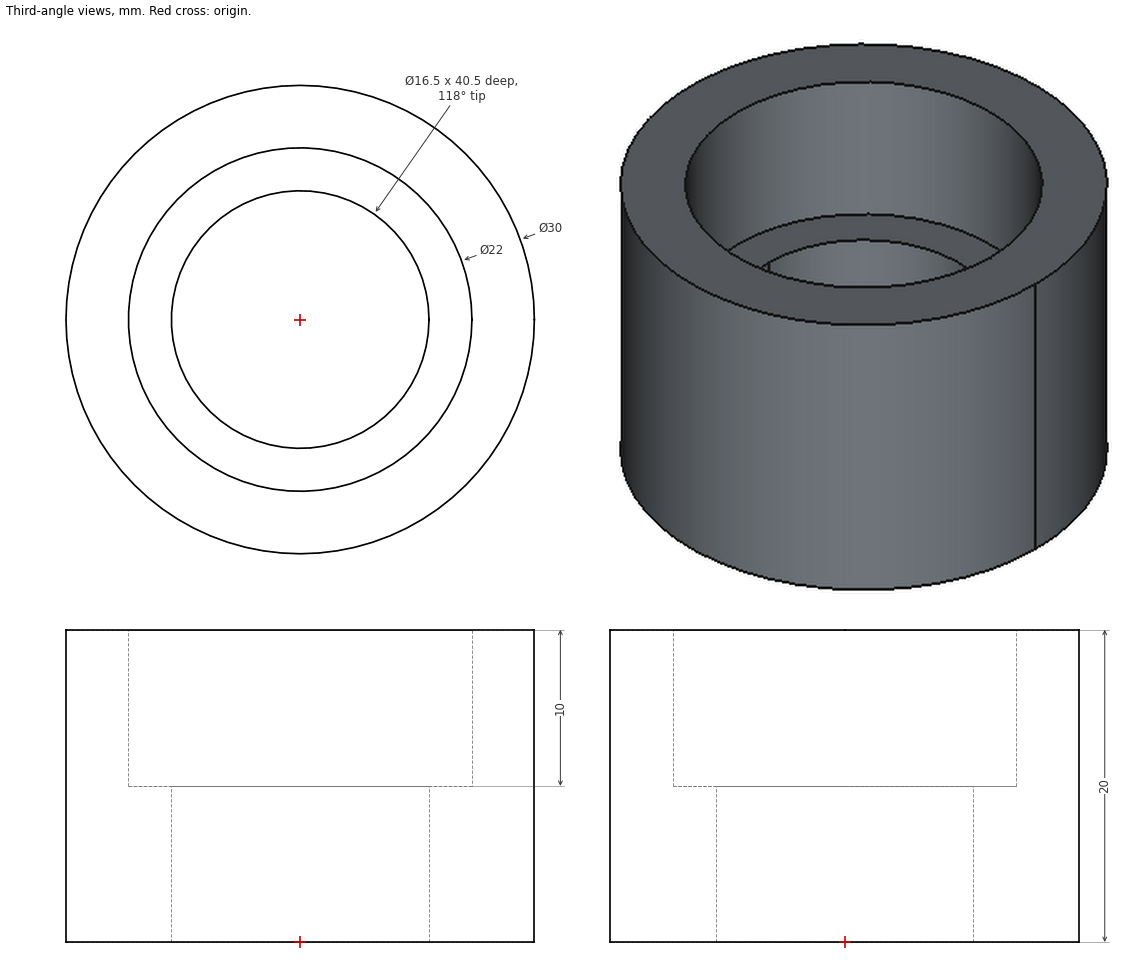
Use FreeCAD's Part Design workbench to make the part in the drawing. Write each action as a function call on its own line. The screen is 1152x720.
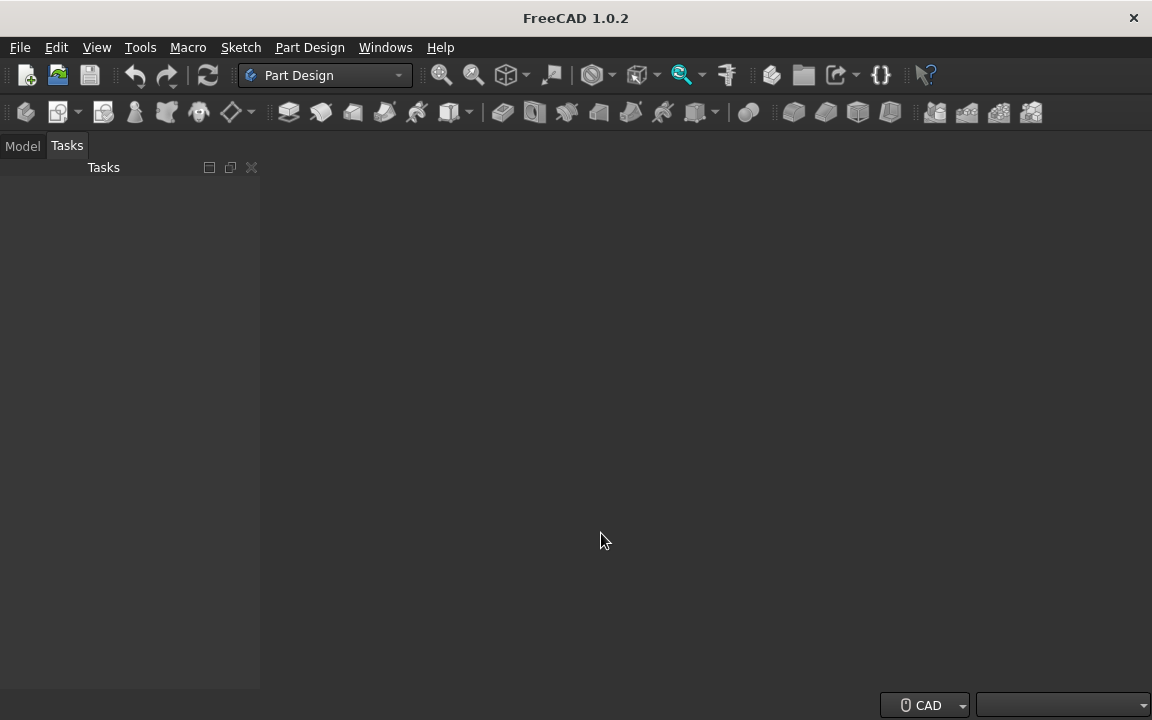
click(26, 76)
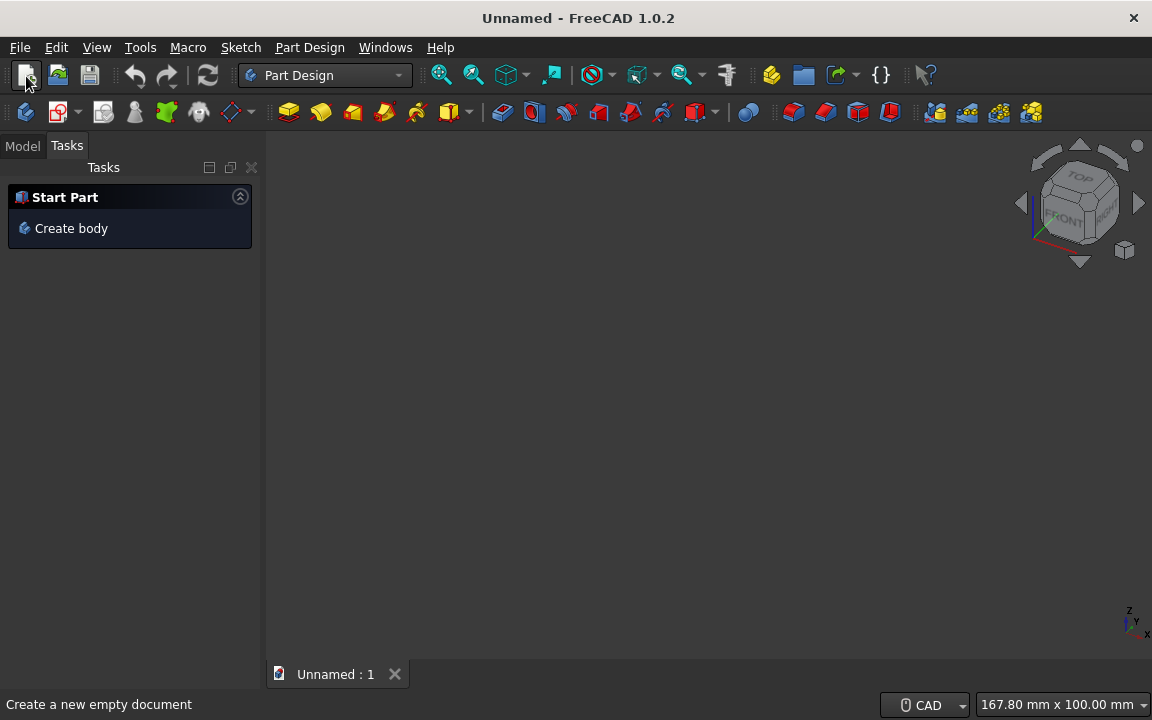
click(58, 112)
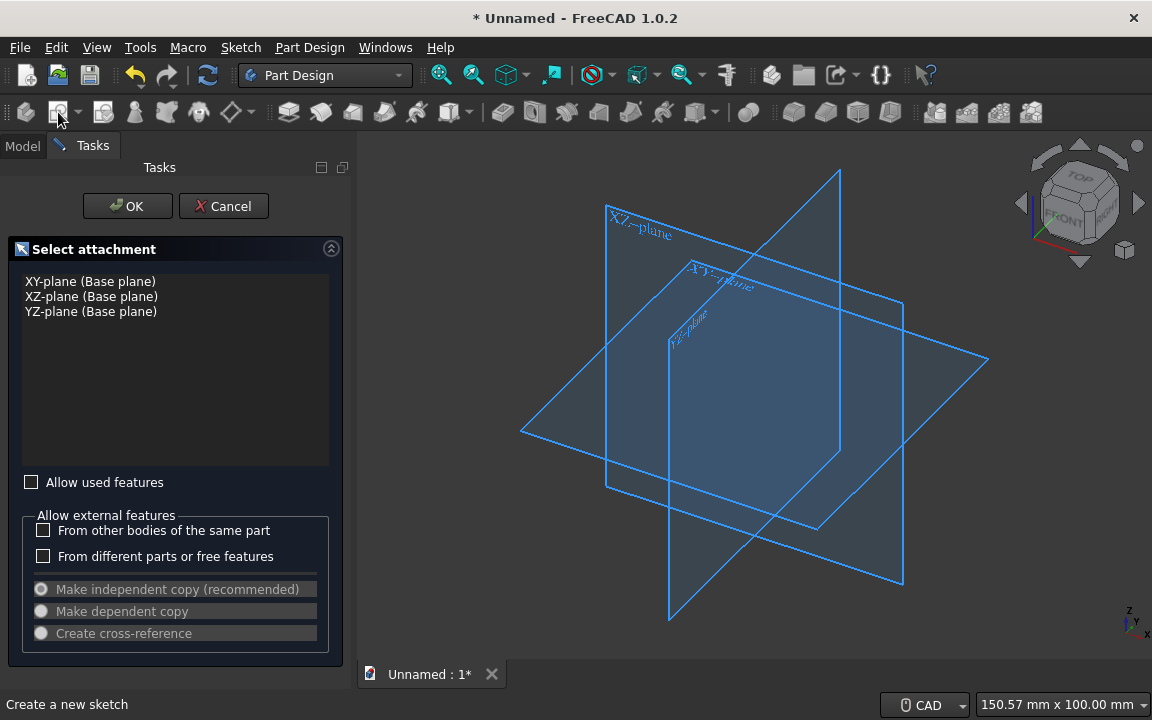
click(82, 282)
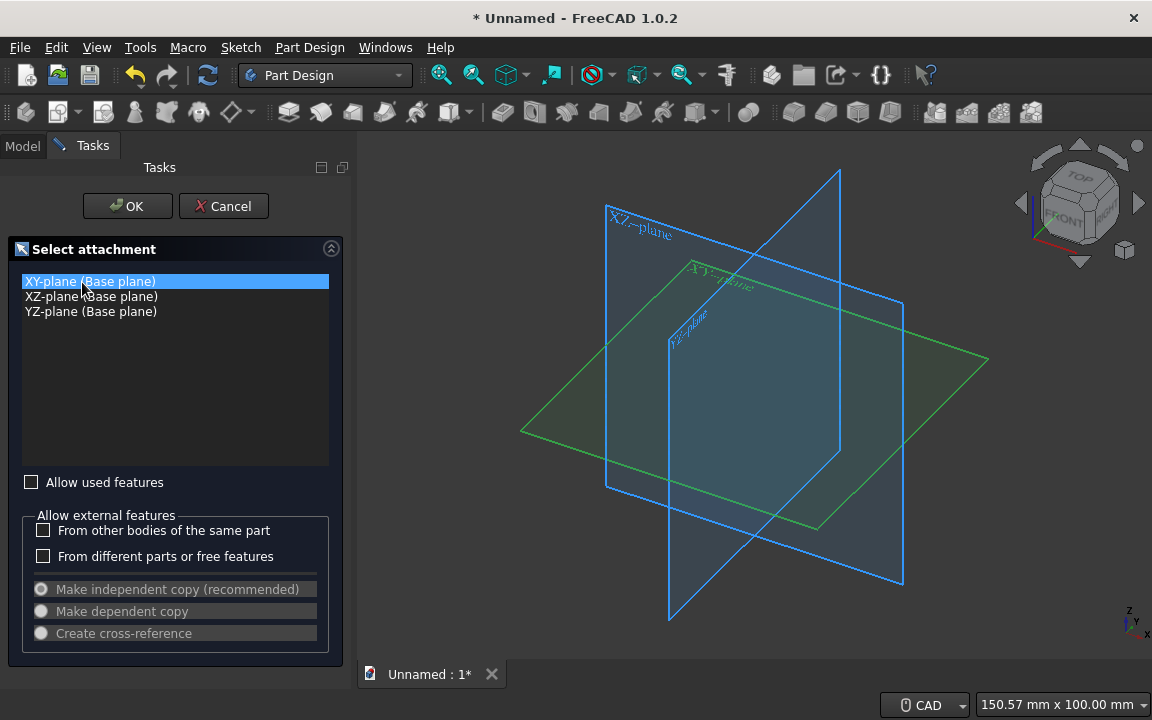
click(128, 206)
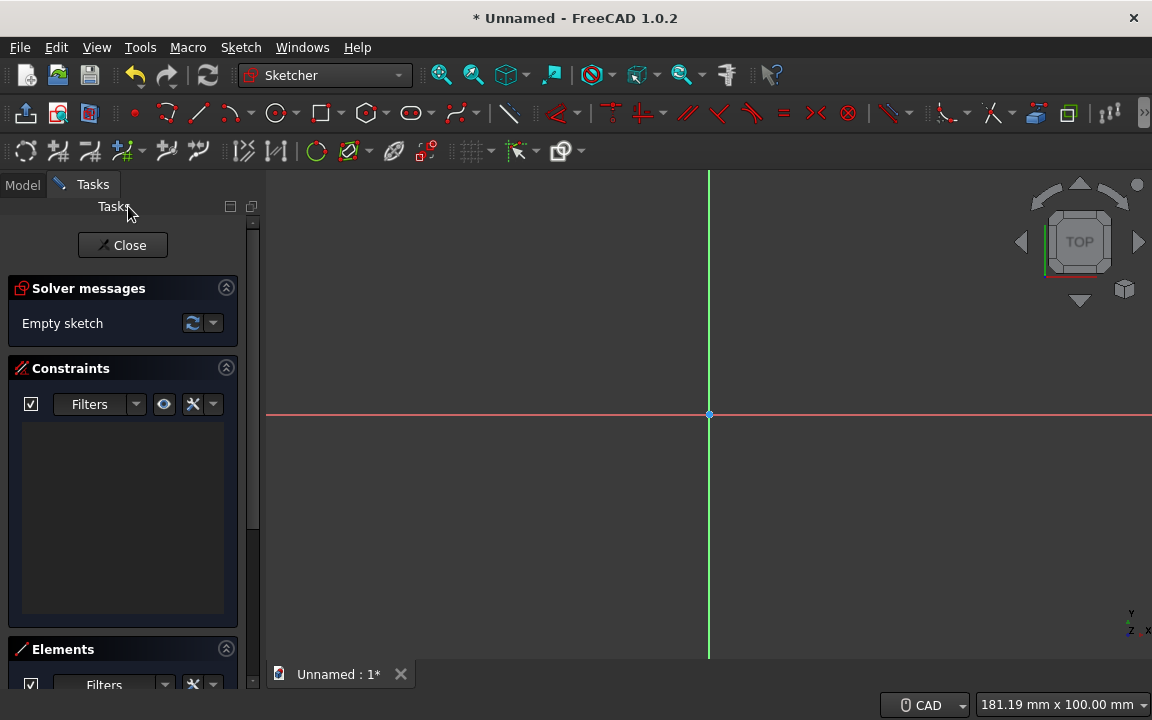
scroll(765, 414, up, 4)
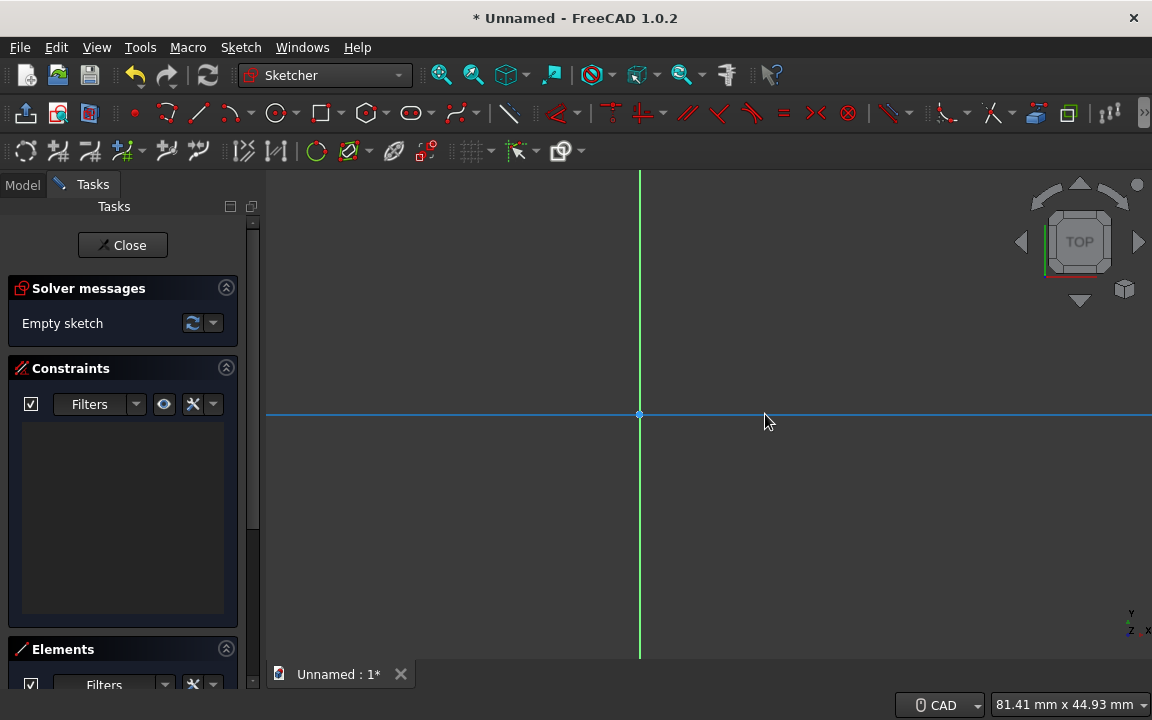
click(276, 114)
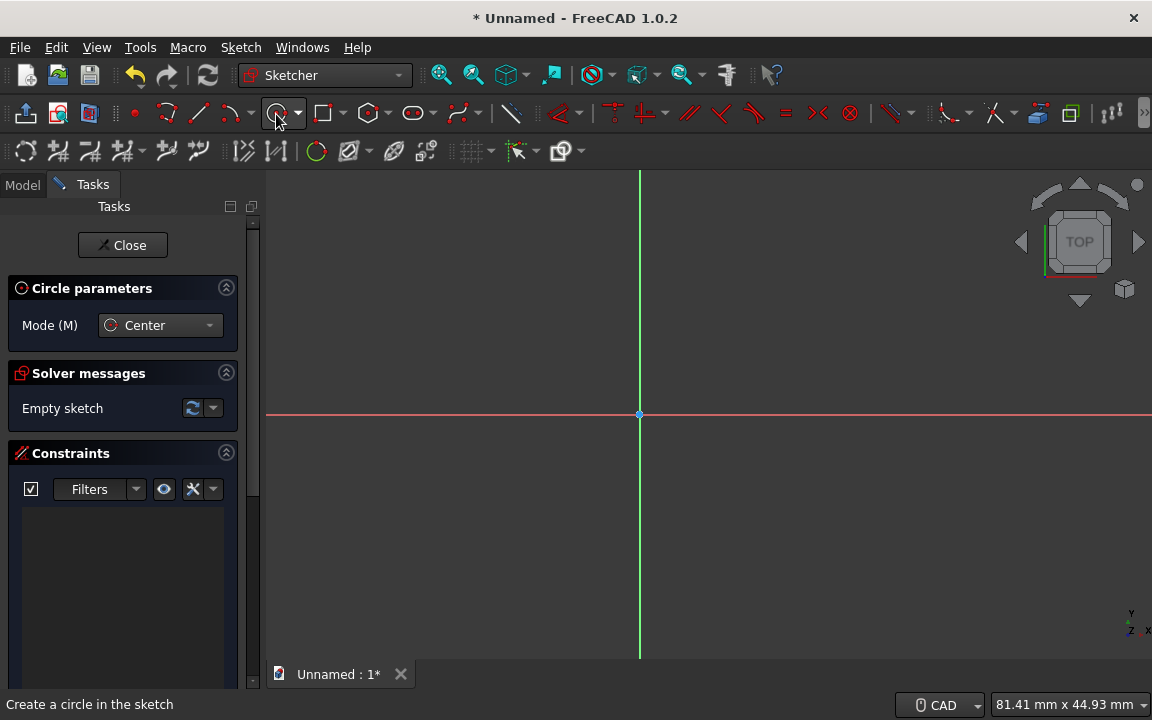
click(640, 414)
click(755, 299)
key(Escape)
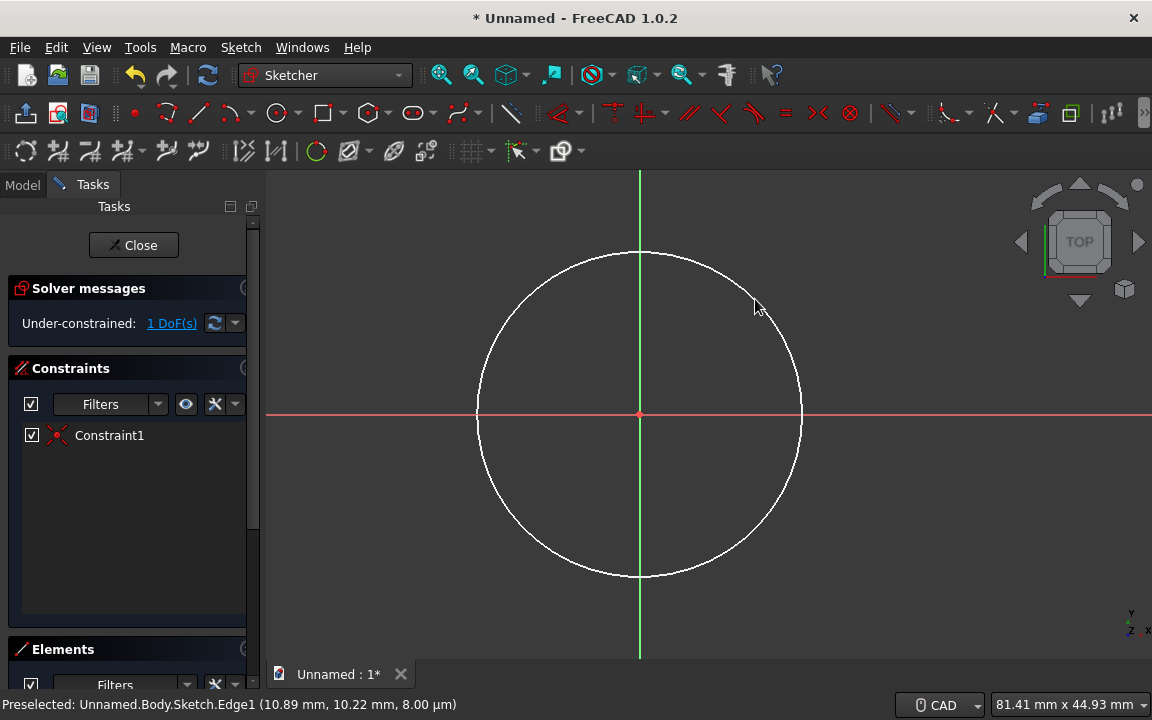
click(558, 114)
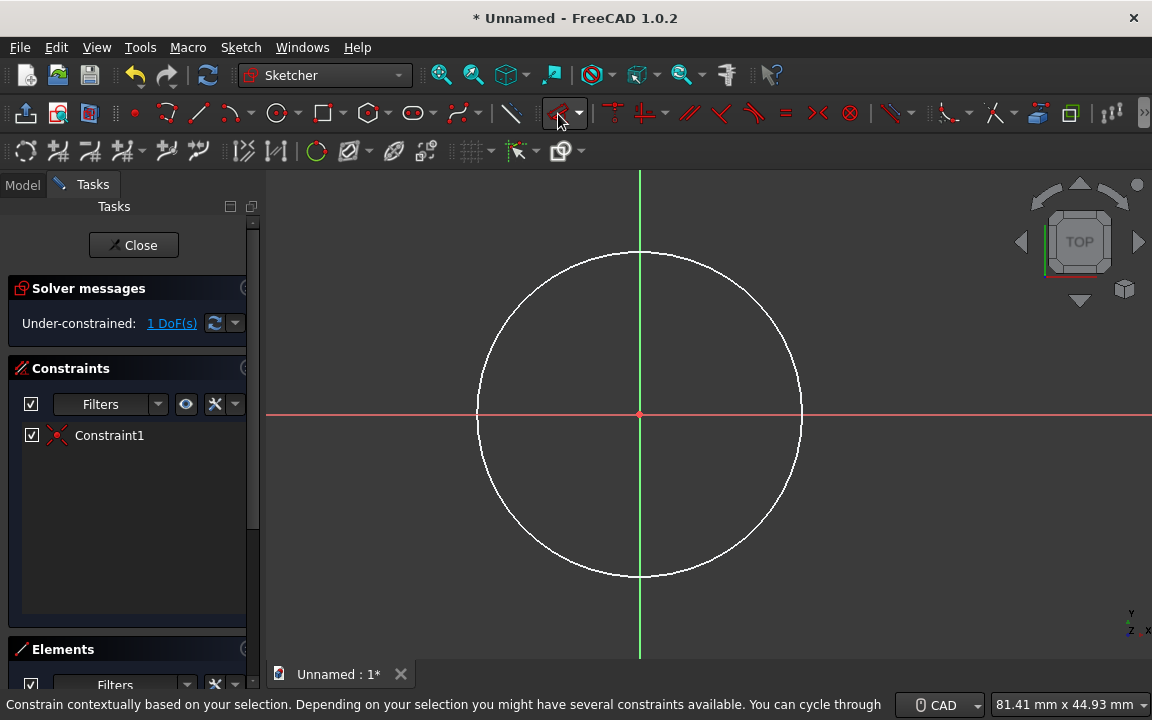
click(754, 299)
click(777, 276)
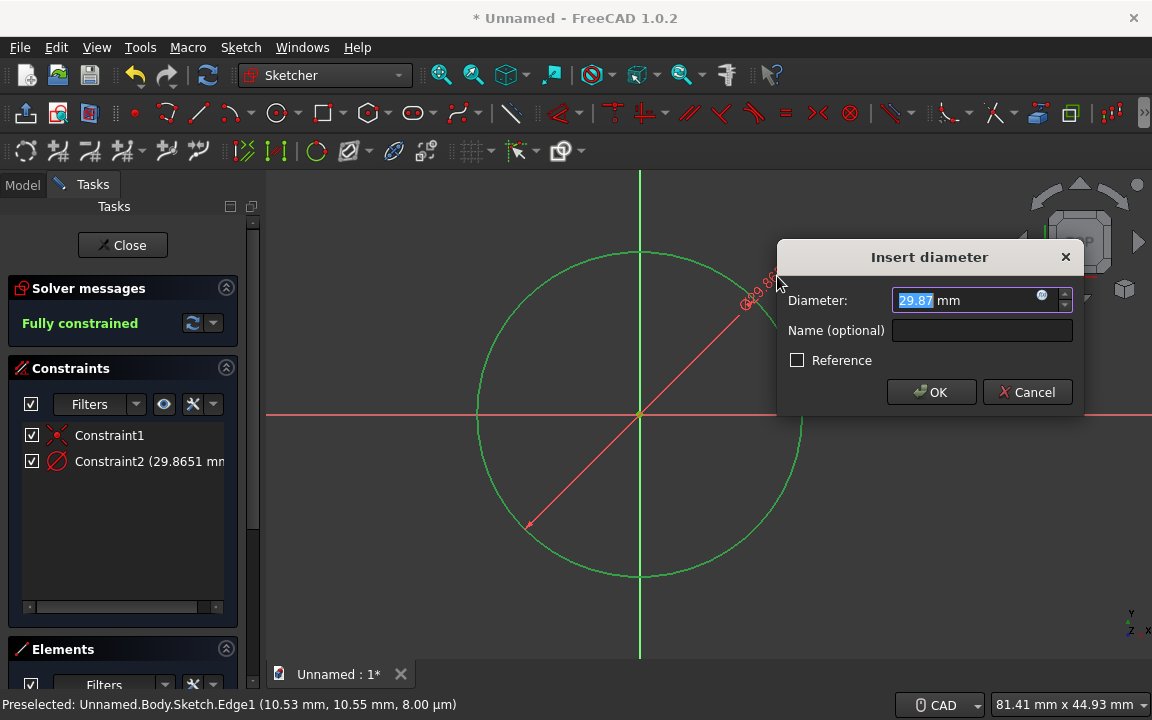
text(30)
key(Return)
key(Escape)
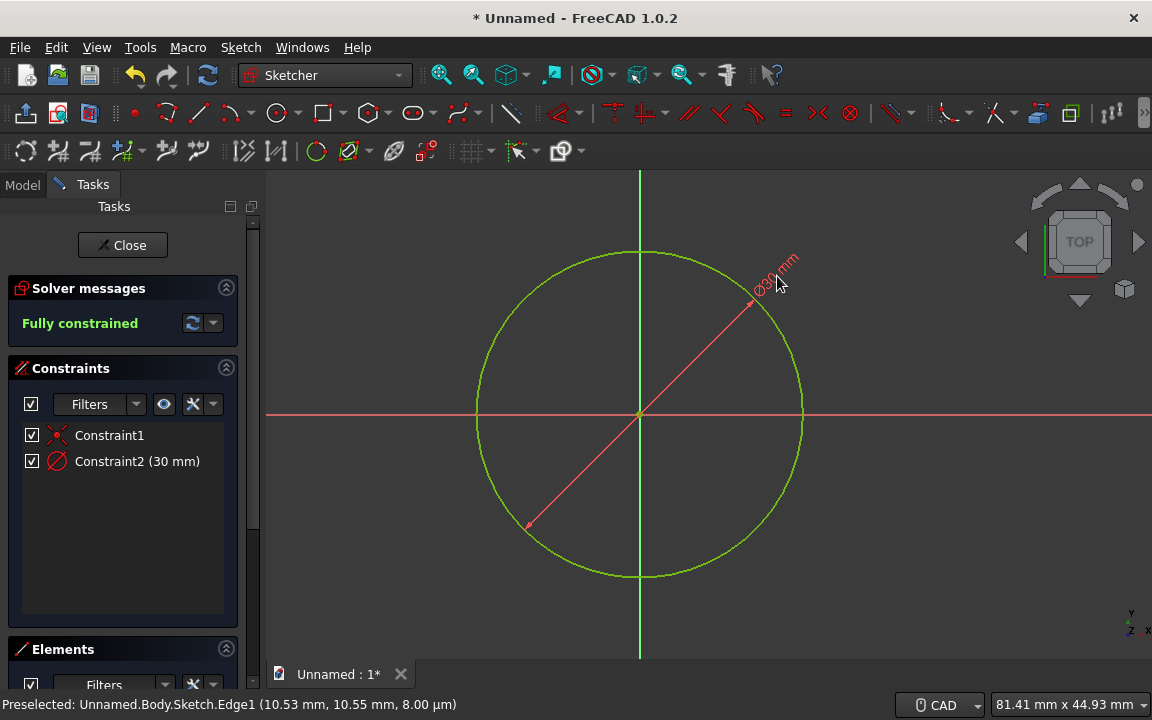
click(123, 245)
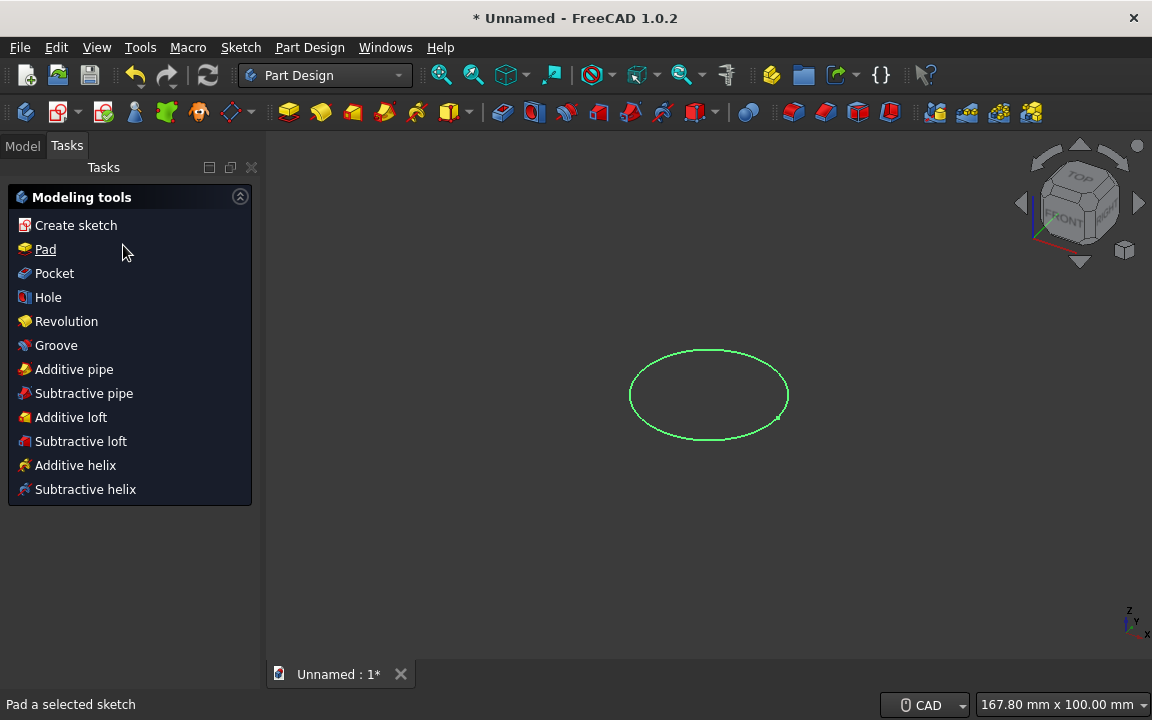
click(290, 112)